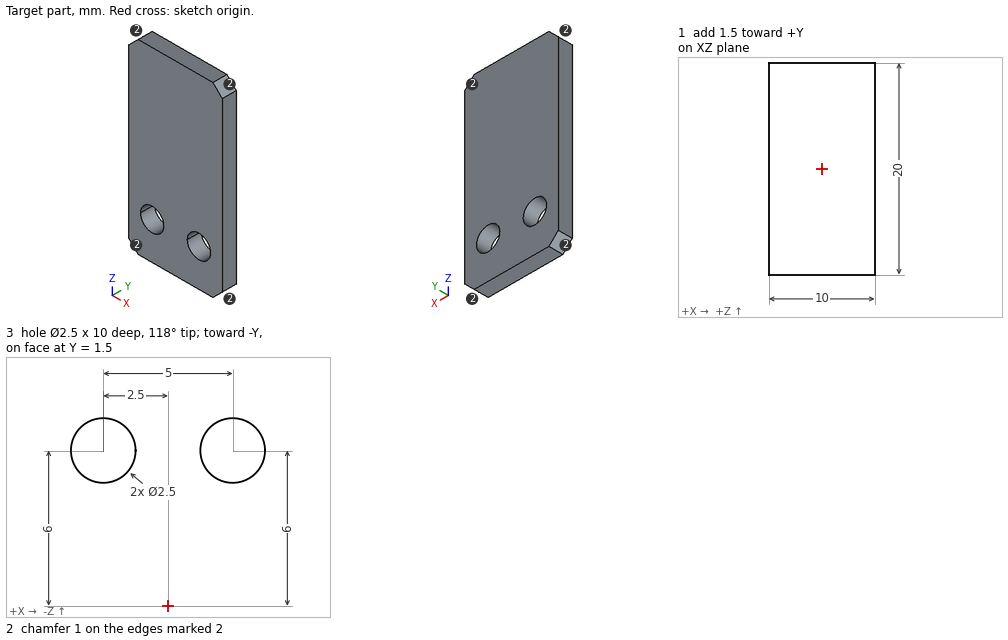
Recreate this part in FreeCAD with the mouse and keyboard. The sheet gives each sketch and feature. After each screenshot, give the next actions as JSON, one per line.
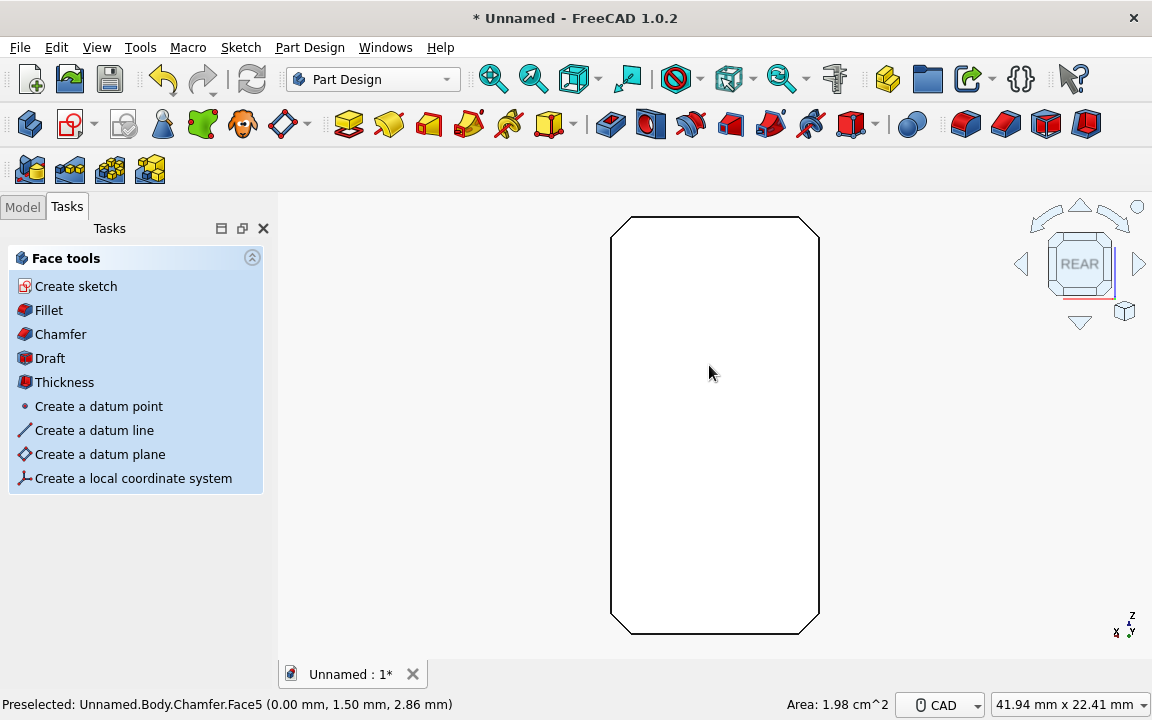
{"action": "left_click", "coordinate": [70, 124]}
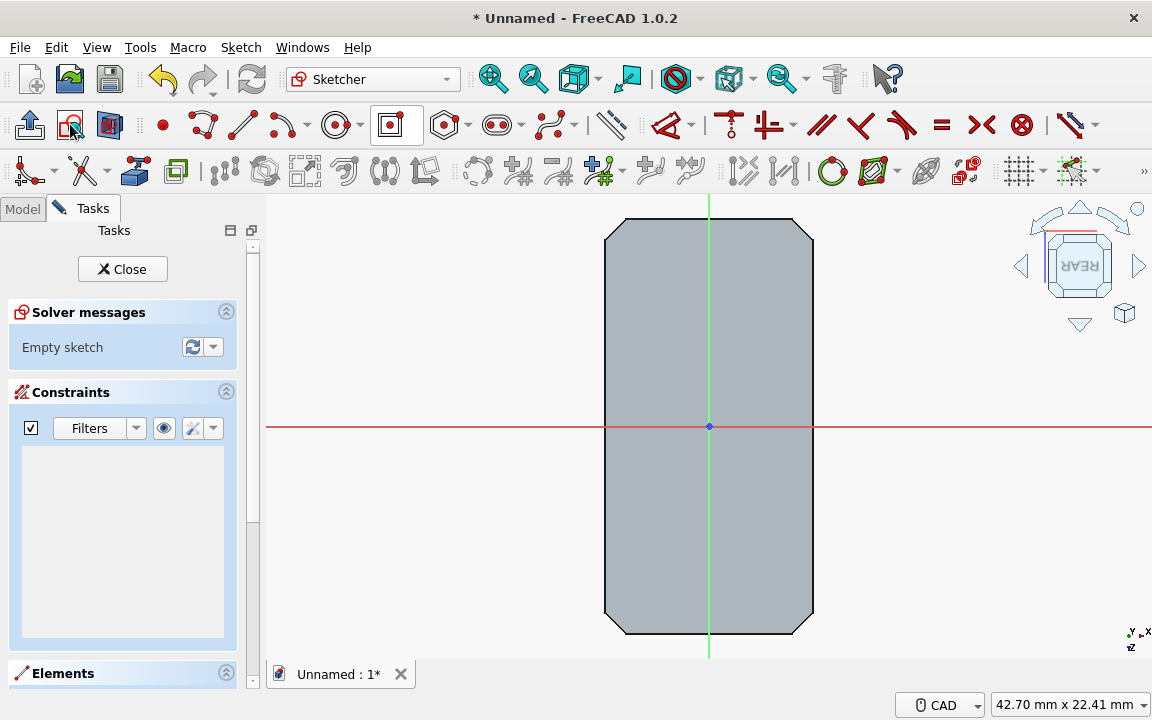
{"action": "scroll", "coordinate": [792, 260], "scroll_direction": "up", "scroll_amount": 3}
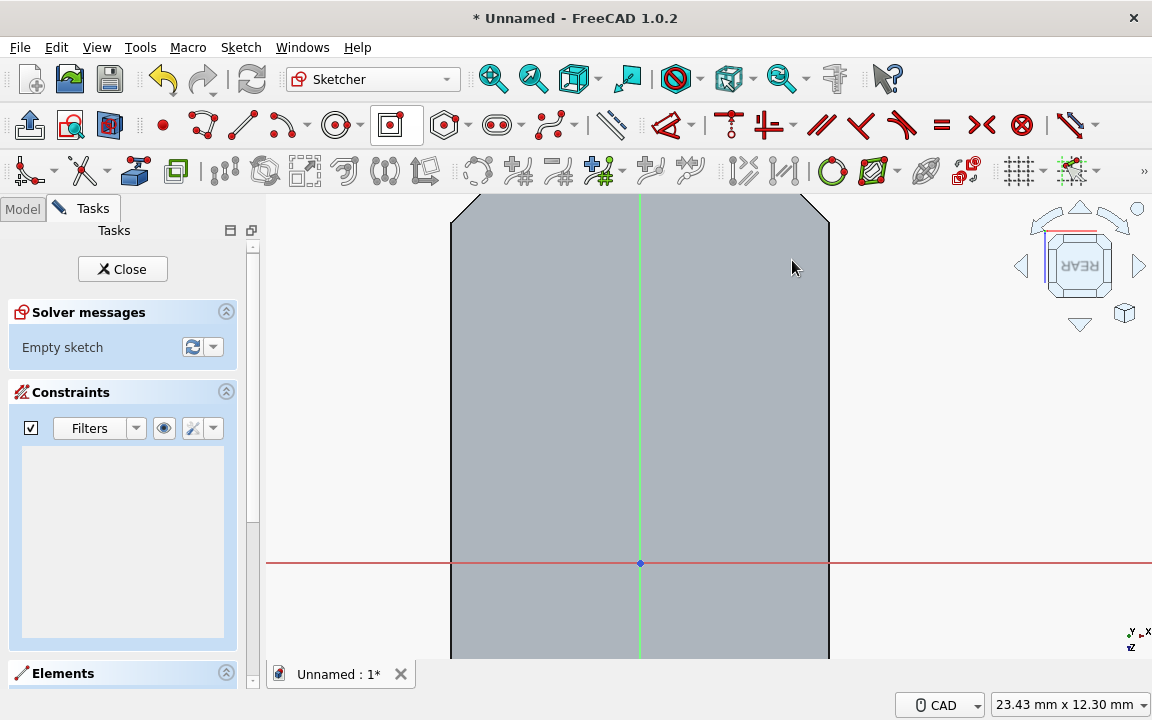
{"action": "key", "text": "g c"}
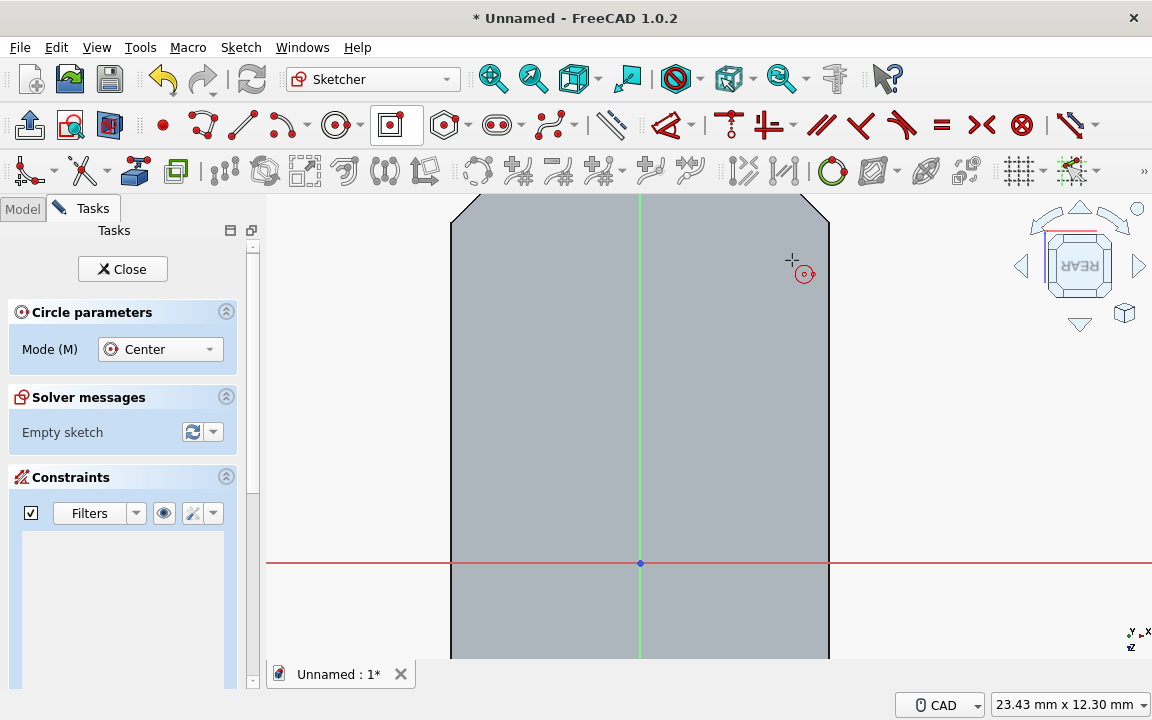
{"action": "left_click", "coordinate": [546, 336]}
{"action": "left_click", "coordinate": [579, 303]}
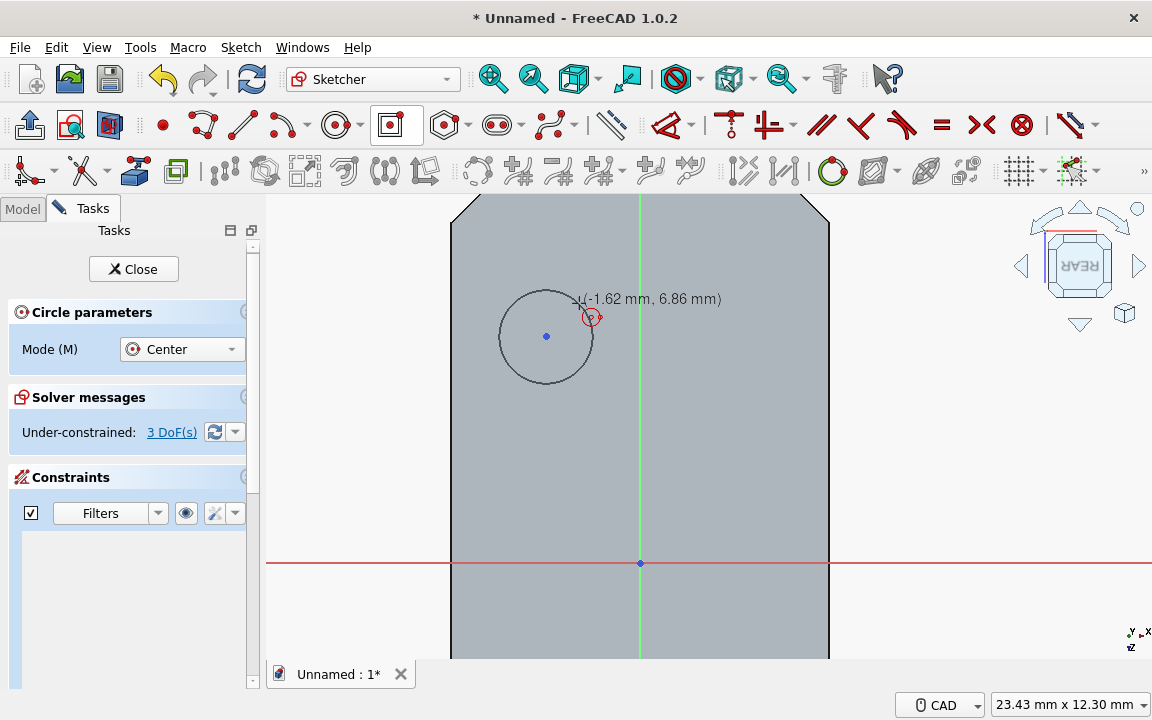
{"action": "left_click", "coordinate": [735, 336]}
{"action": "left_click", "coordinate": [768, 303]}
{"action": "key", "text": "Escape"}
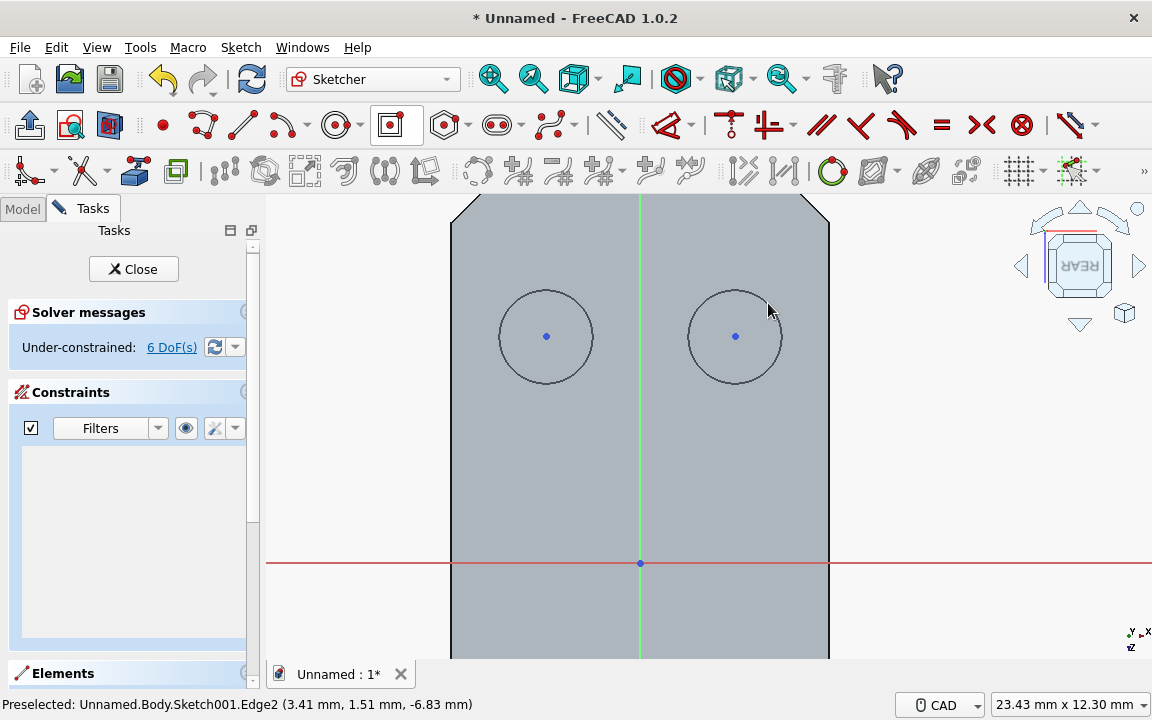
{"action": "left_click", "coordinate": [579, 304]}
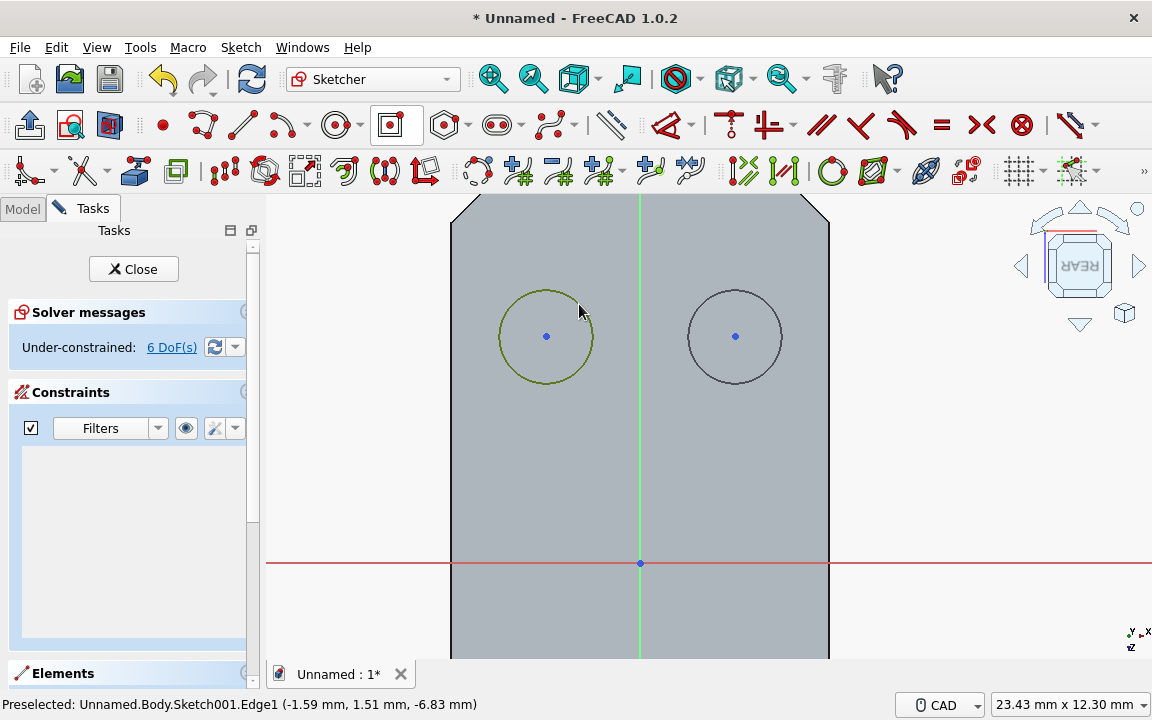
{"action": "left_click", "coordinate": [768, 304]}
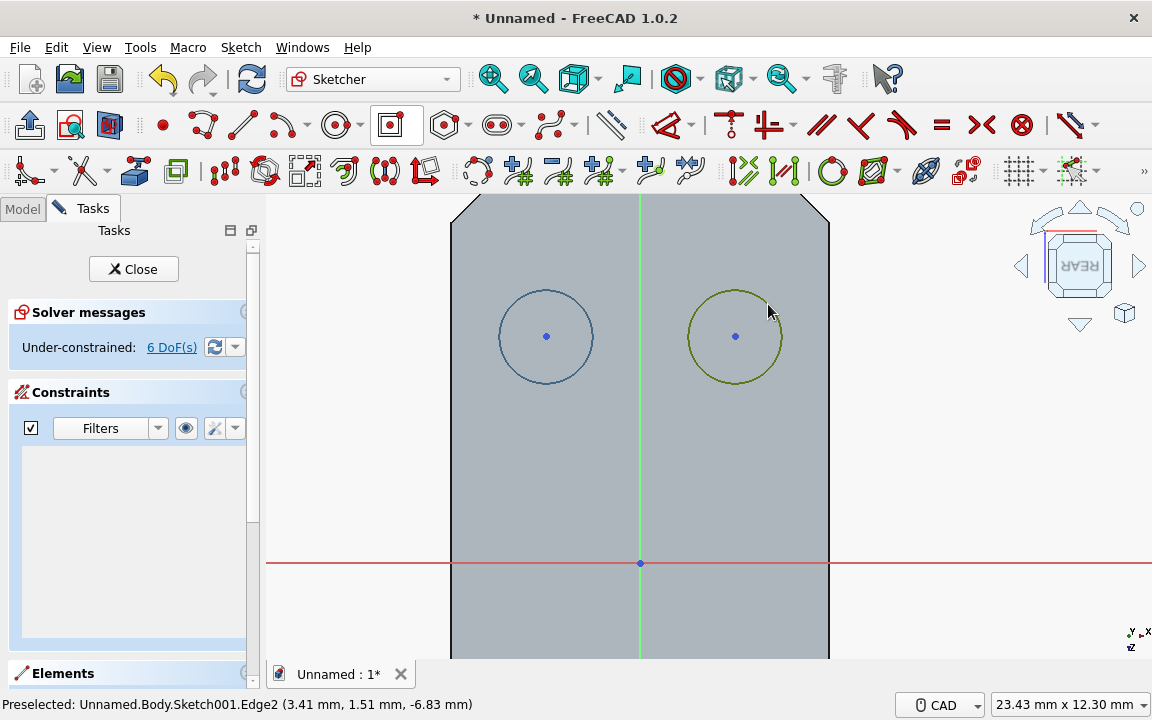
{"action": "left_click", "coordinate": [942, 126]}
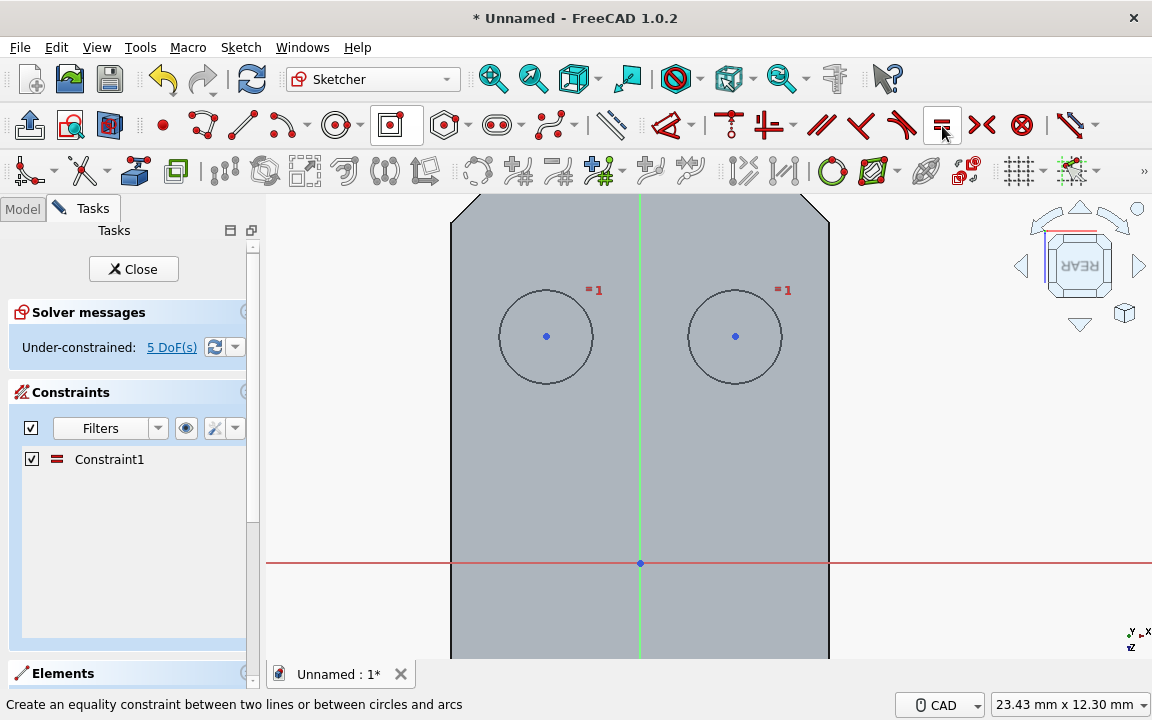
{"action": "left_click", "coordinate": [666, 126]}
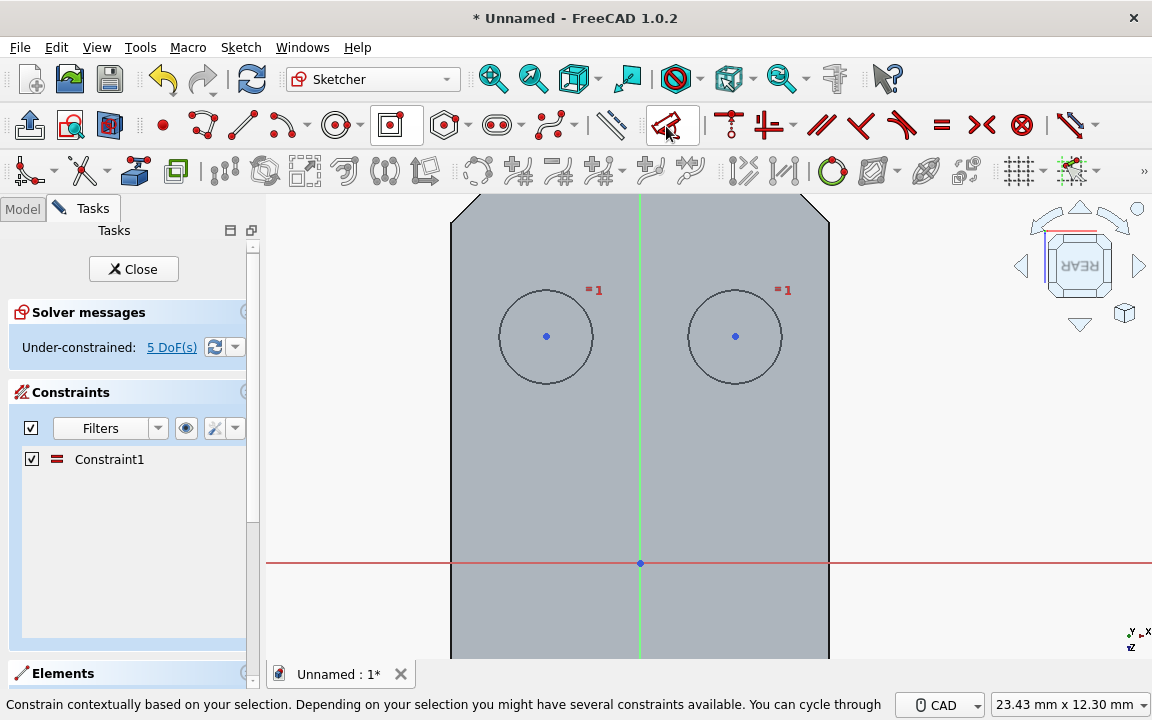
{"action": "left_click", "coordinate": [579, 304]}
{"action": "left_click", "coordinate": [602, 281]}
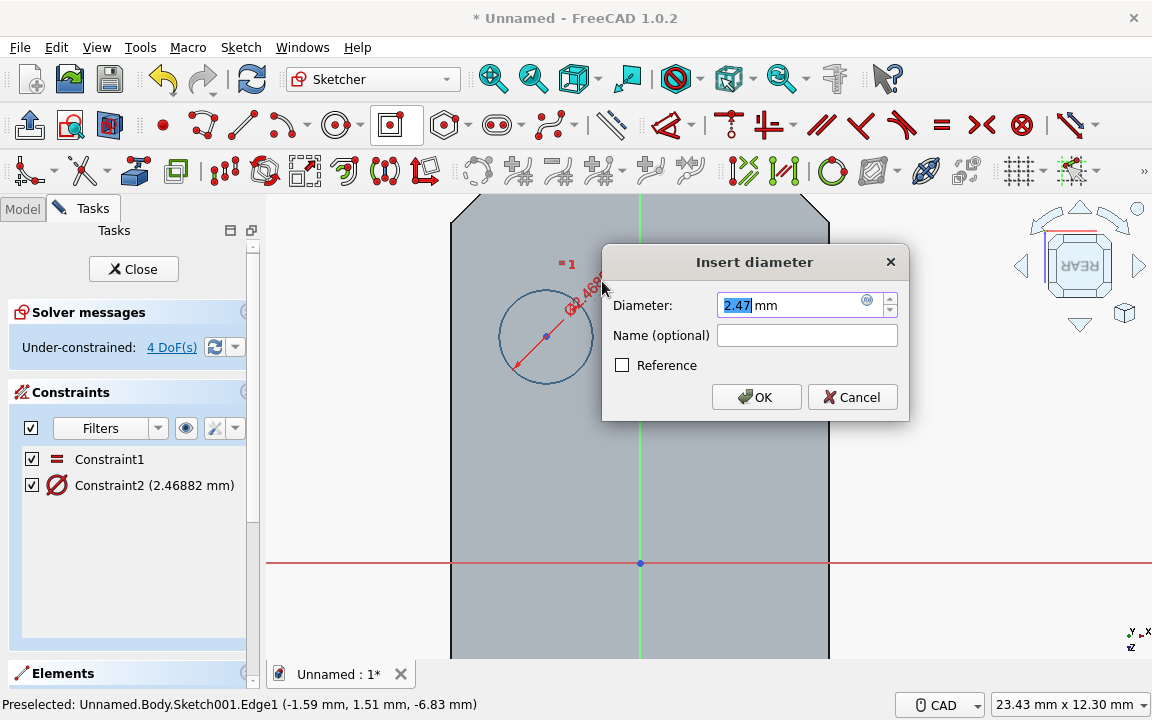
{"action": "type", "text": "2.5"}
{"action": "key", "text": "Return"}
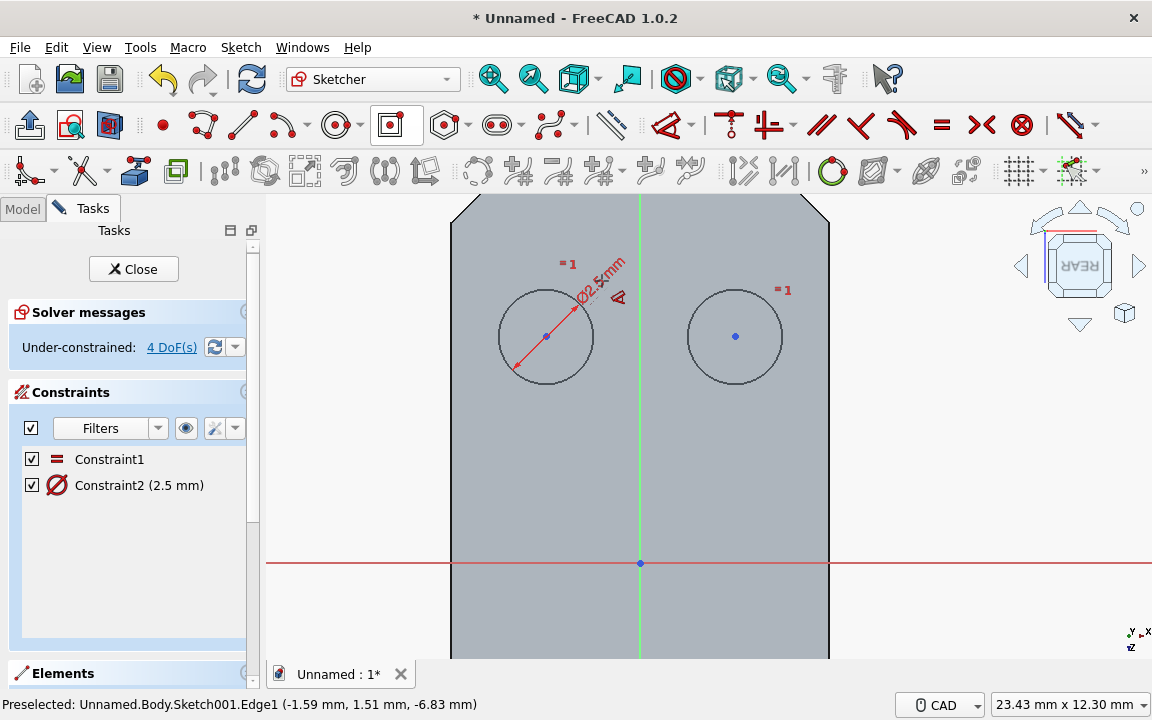
{"action": "left_click", "coordinate": [546, 337]}
{"action": "left_click", "coordinate": [512, 450]}